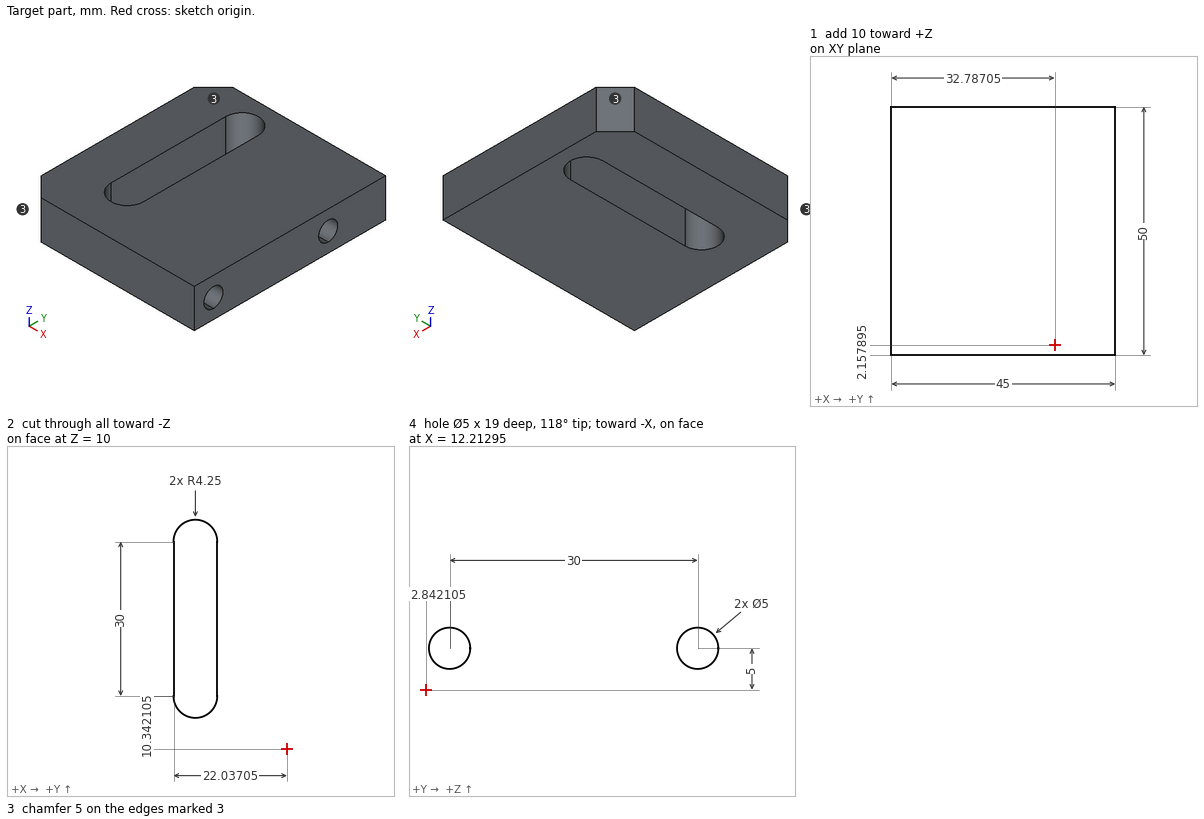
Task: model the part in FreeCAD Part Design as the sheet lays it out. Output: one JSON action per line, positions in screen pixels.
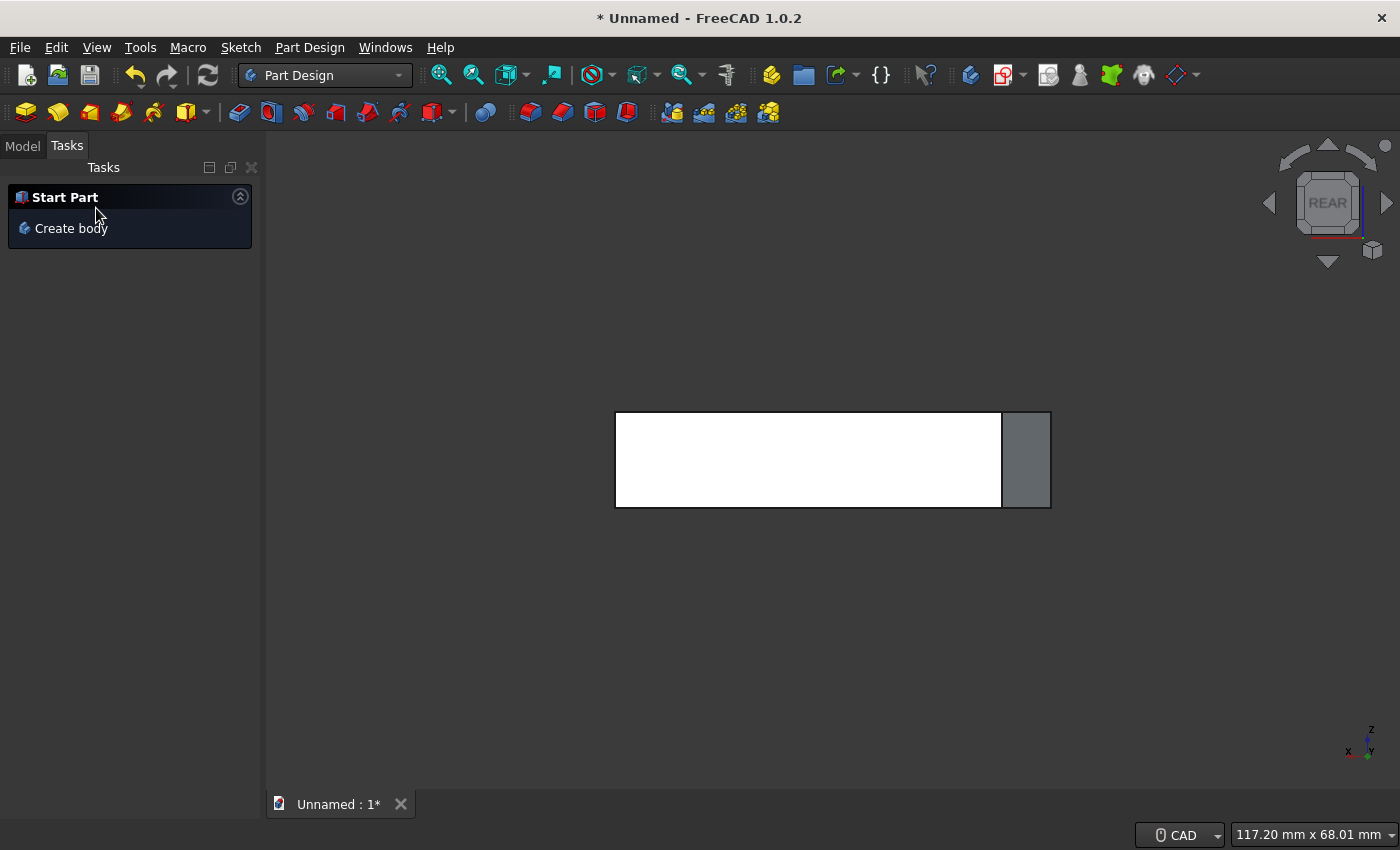
{"action": "key", "text": "0"}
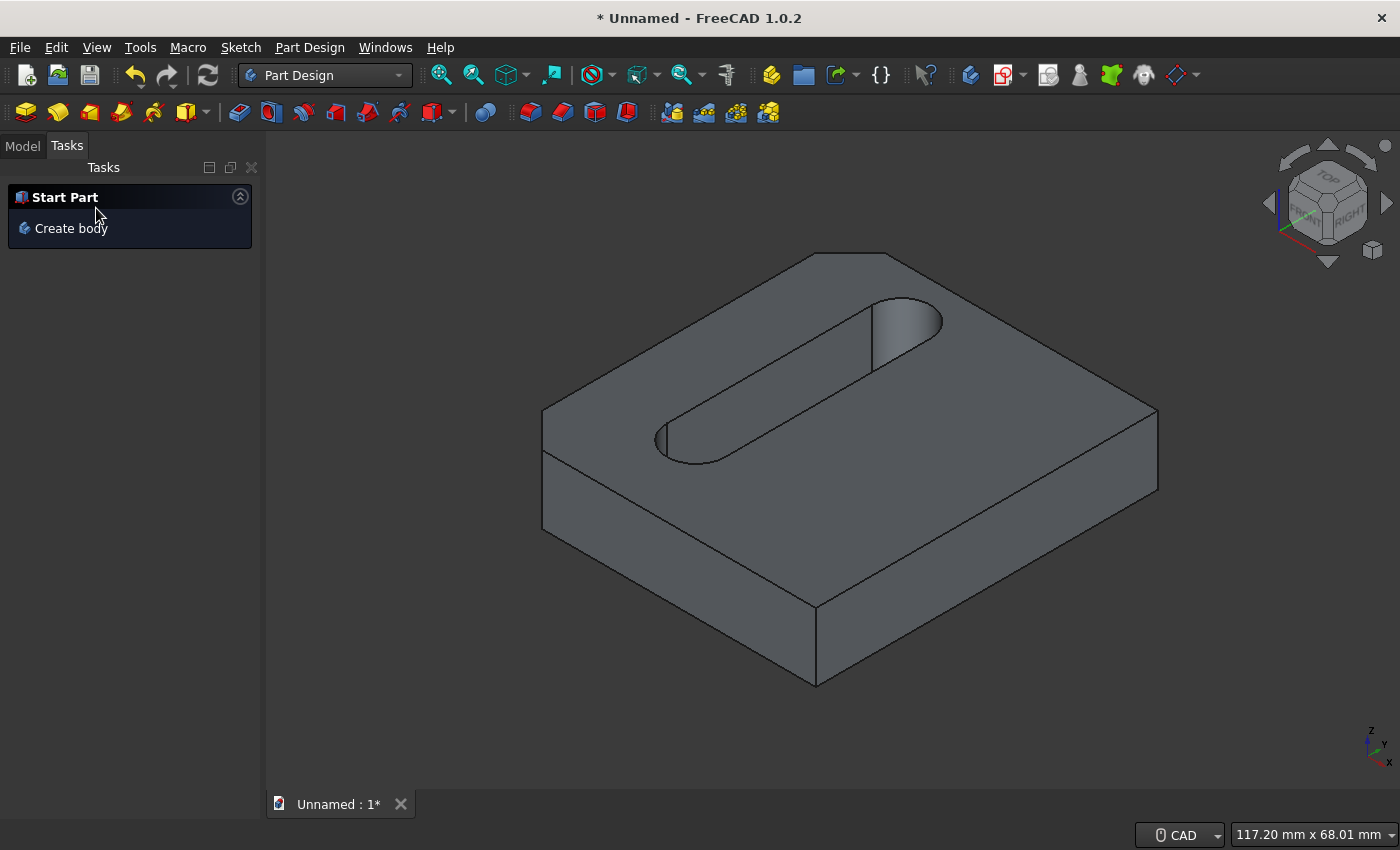
{"action": "left_click", "coordinate": [1085, 491]}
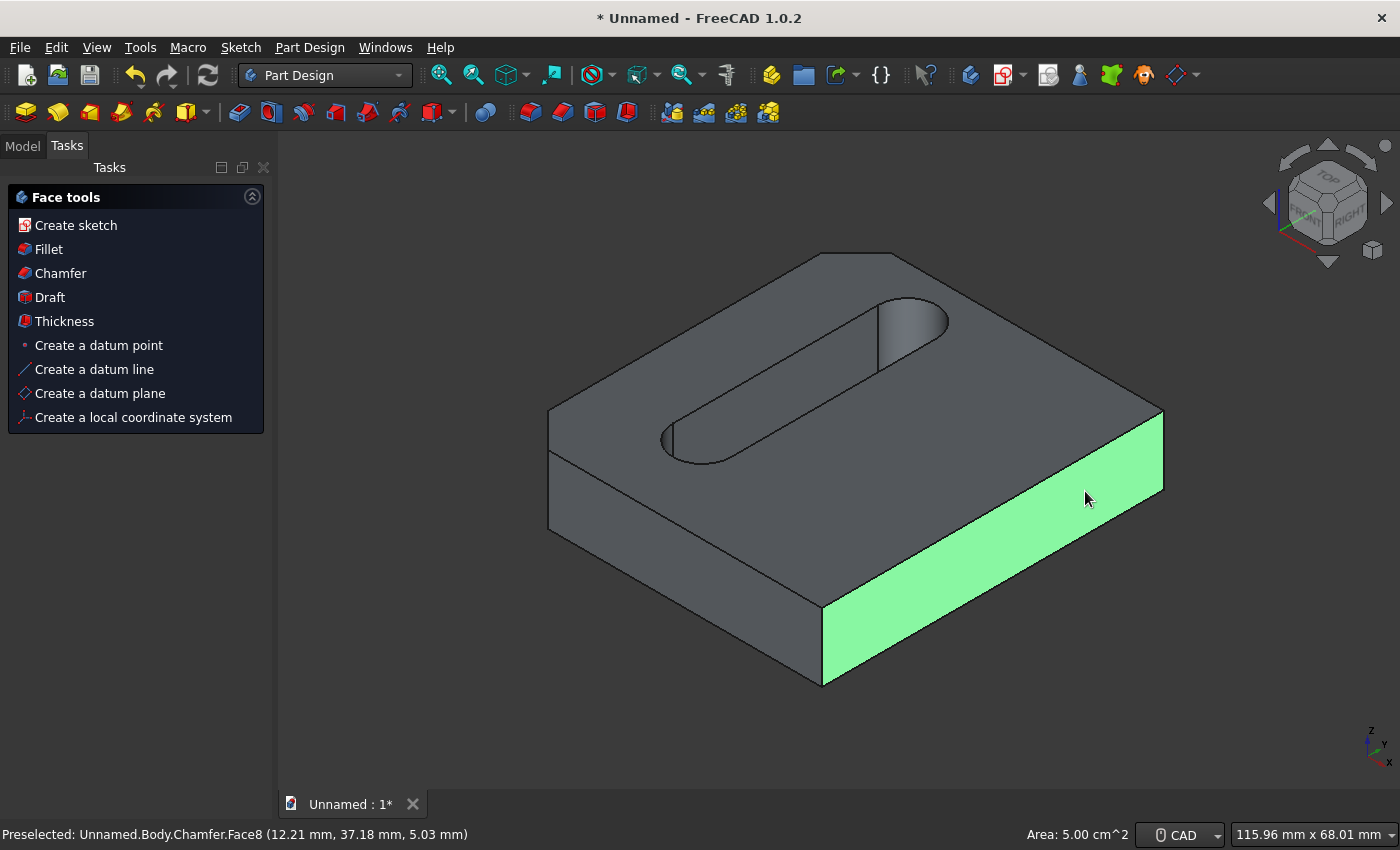
{"action": "left_click", "coordinate": [1004, 76]}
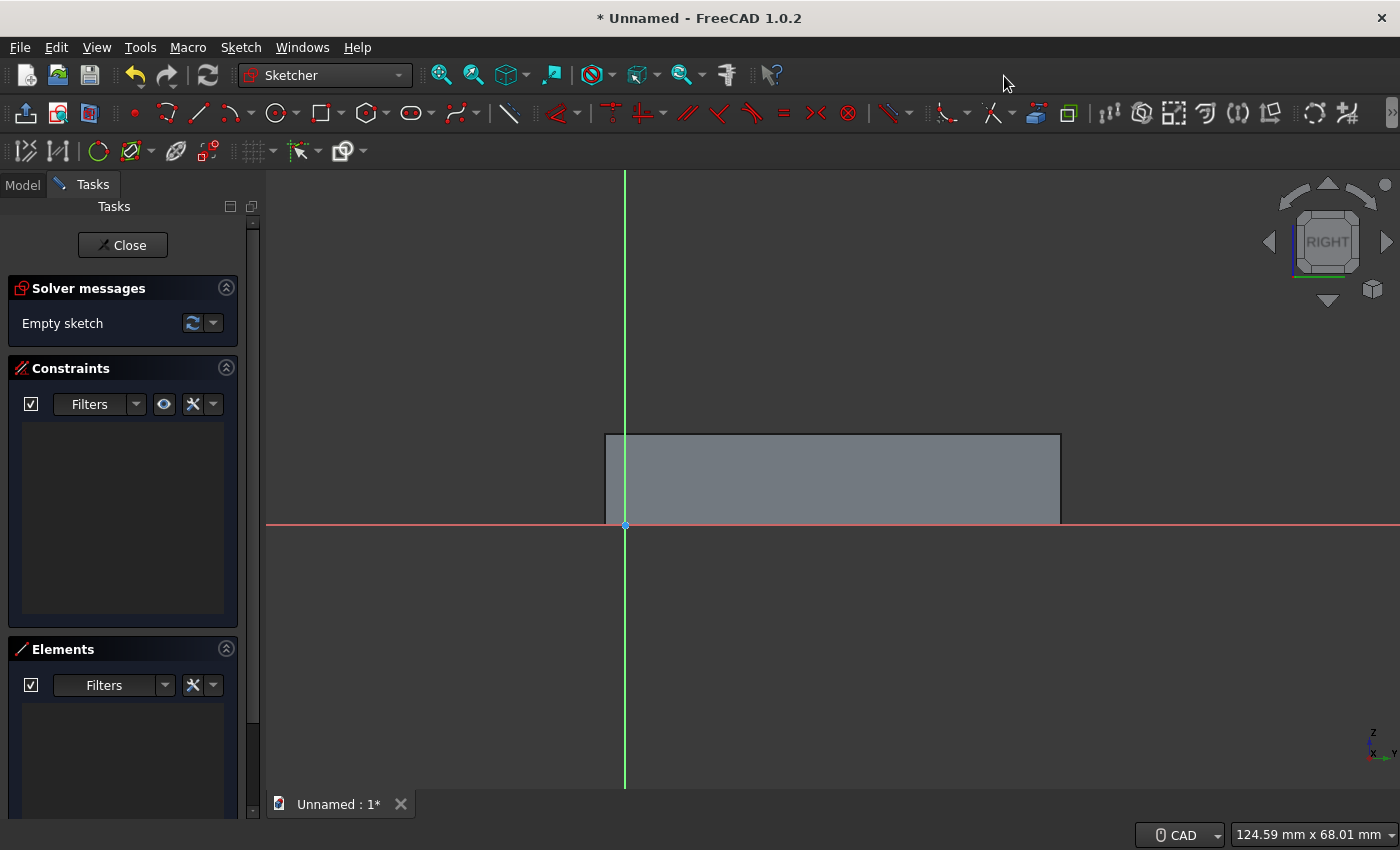
{"action": "scroll", "coordinate": [803, 500], "scroll_direction": "up", "scroll_amount": 4}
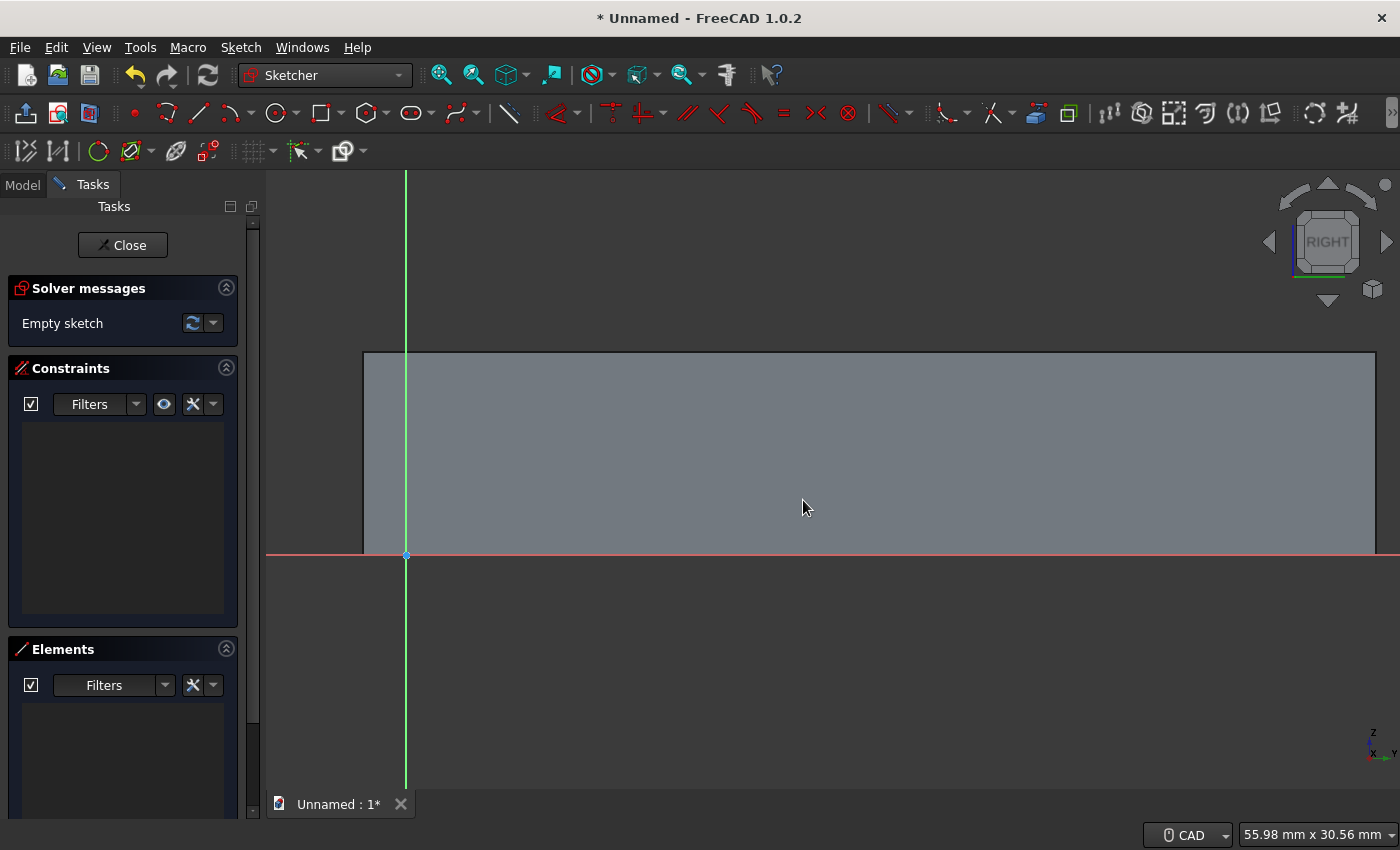
{"action": "left_click", "coordinate": [276, 114]}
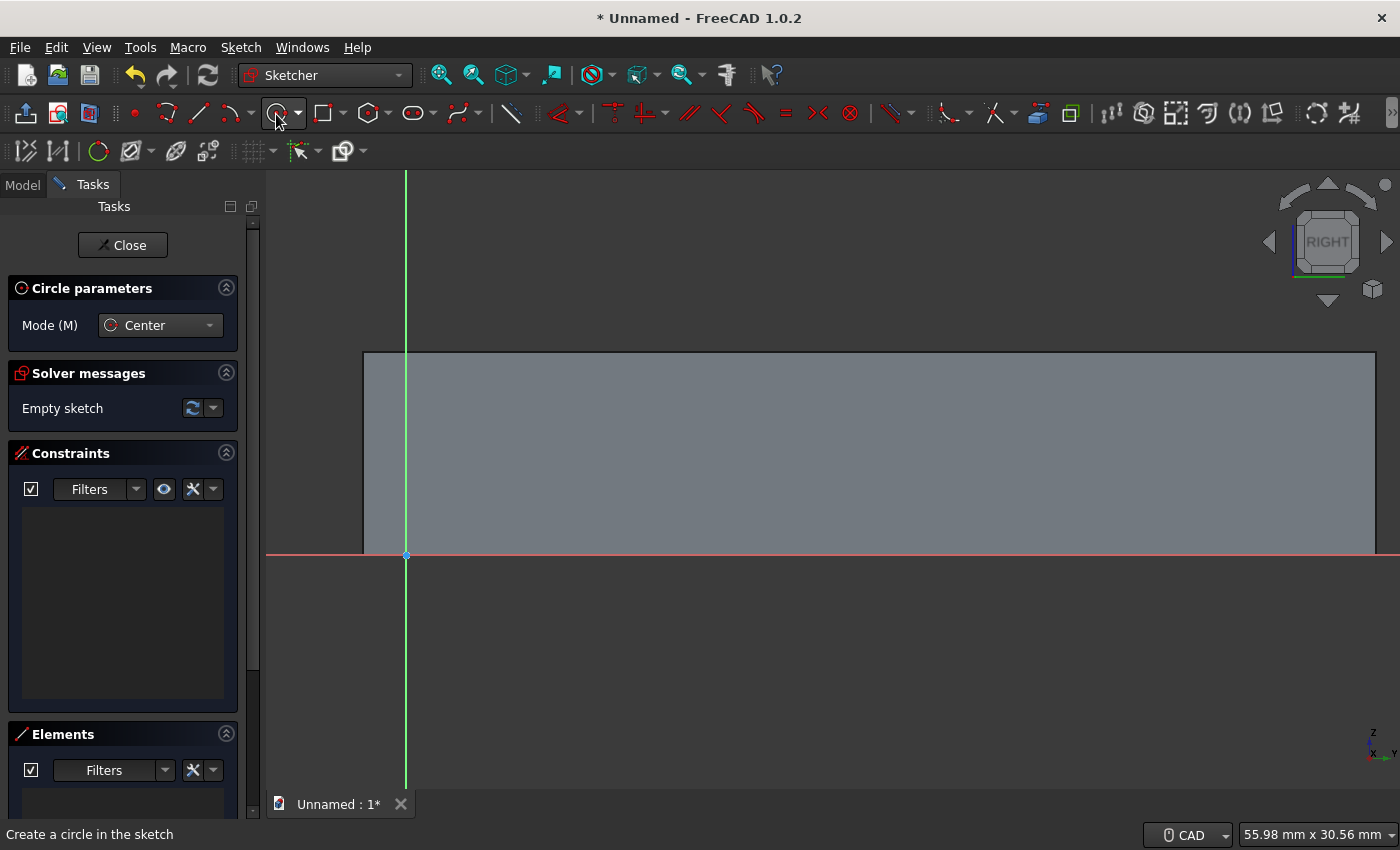
{"action": "left_click", "coordinate": [1072, 454]}
{"action": "mouse_move", "coordinate": [1108, 418]}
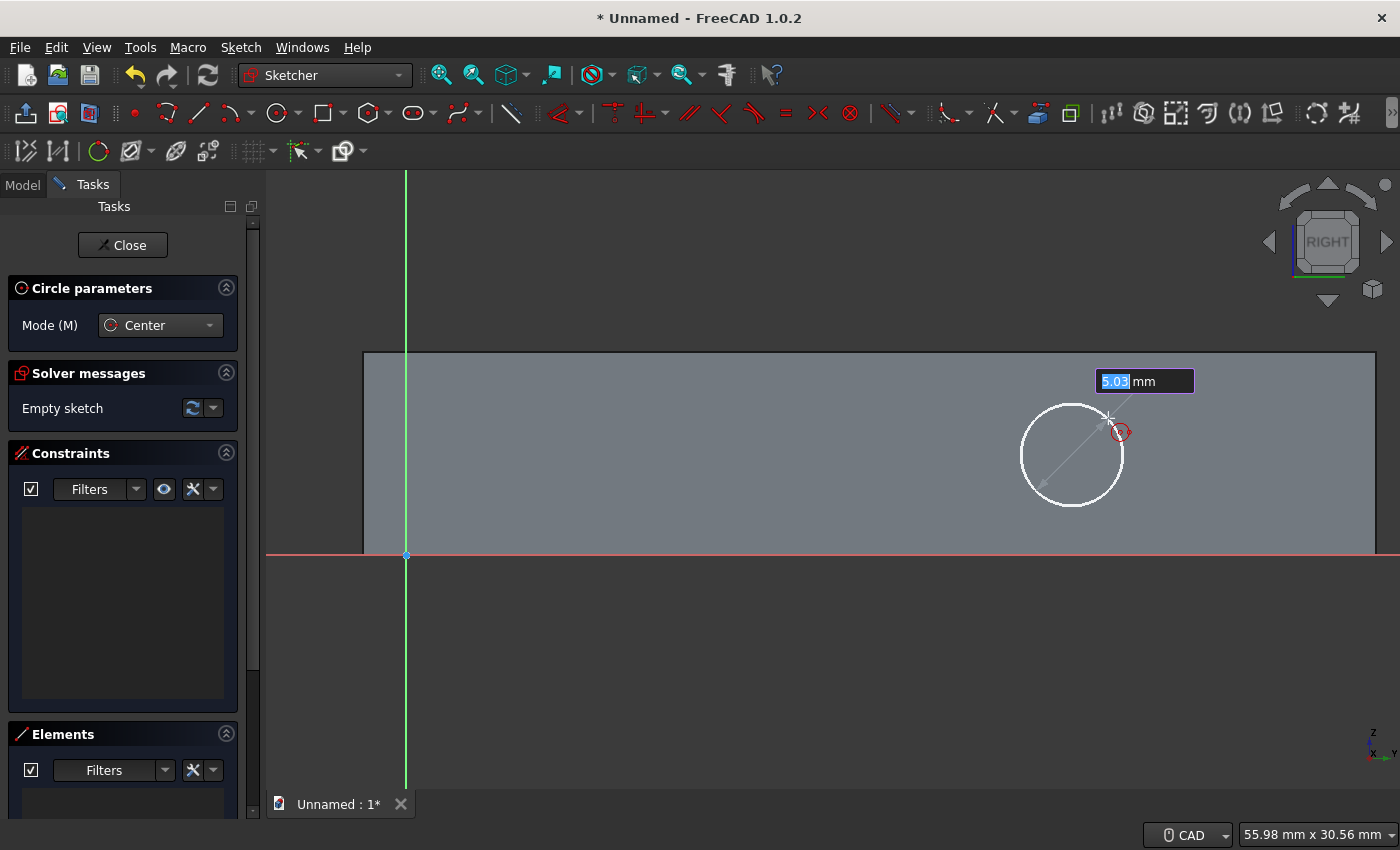
{"action": "type", "text": "5"}
{"action": "key", "text": "Return"}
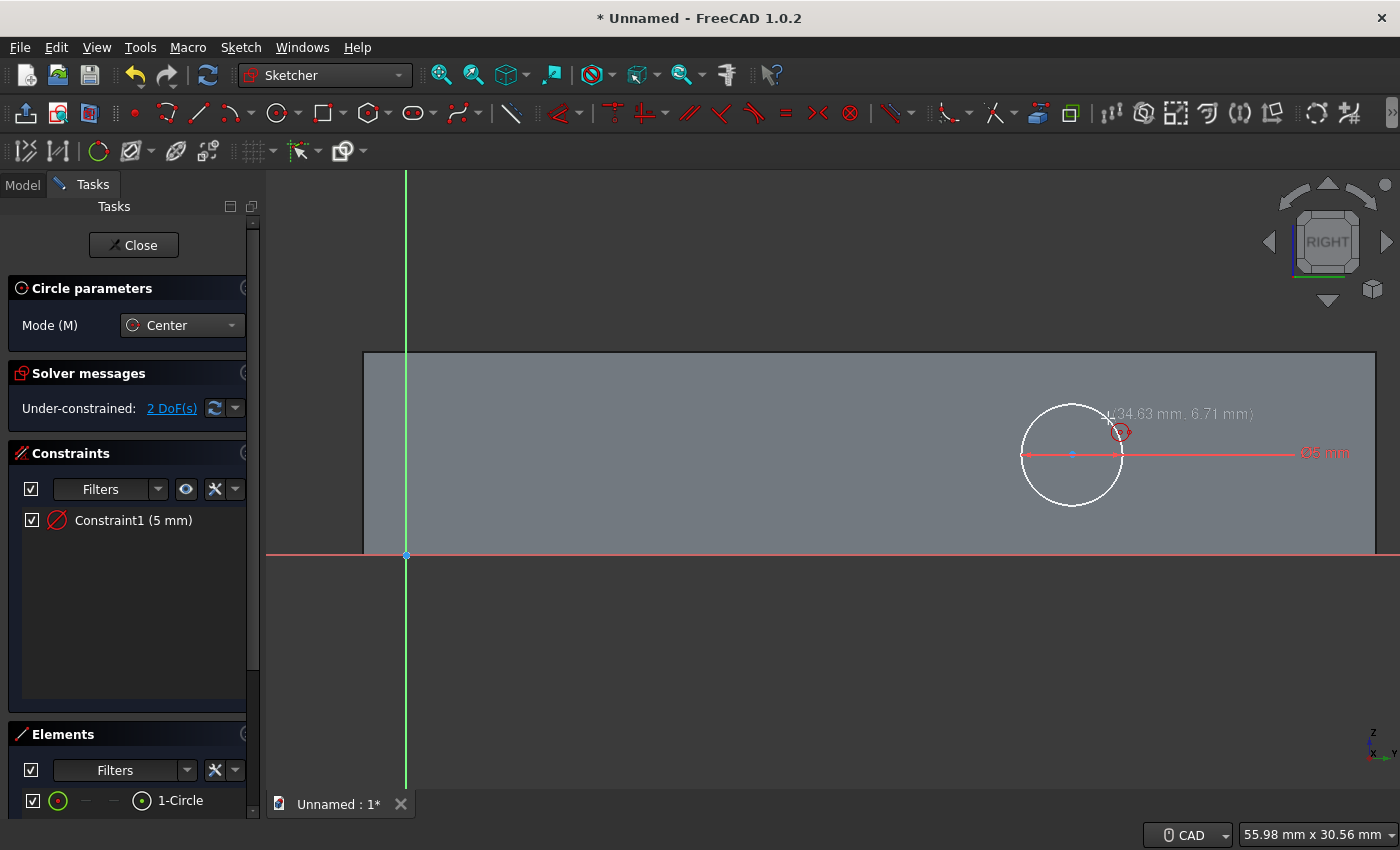
{"action": "left_click", "coordinate": [464, 454]}
{"action": "mouse_move", "coordinate": [500, 418]}